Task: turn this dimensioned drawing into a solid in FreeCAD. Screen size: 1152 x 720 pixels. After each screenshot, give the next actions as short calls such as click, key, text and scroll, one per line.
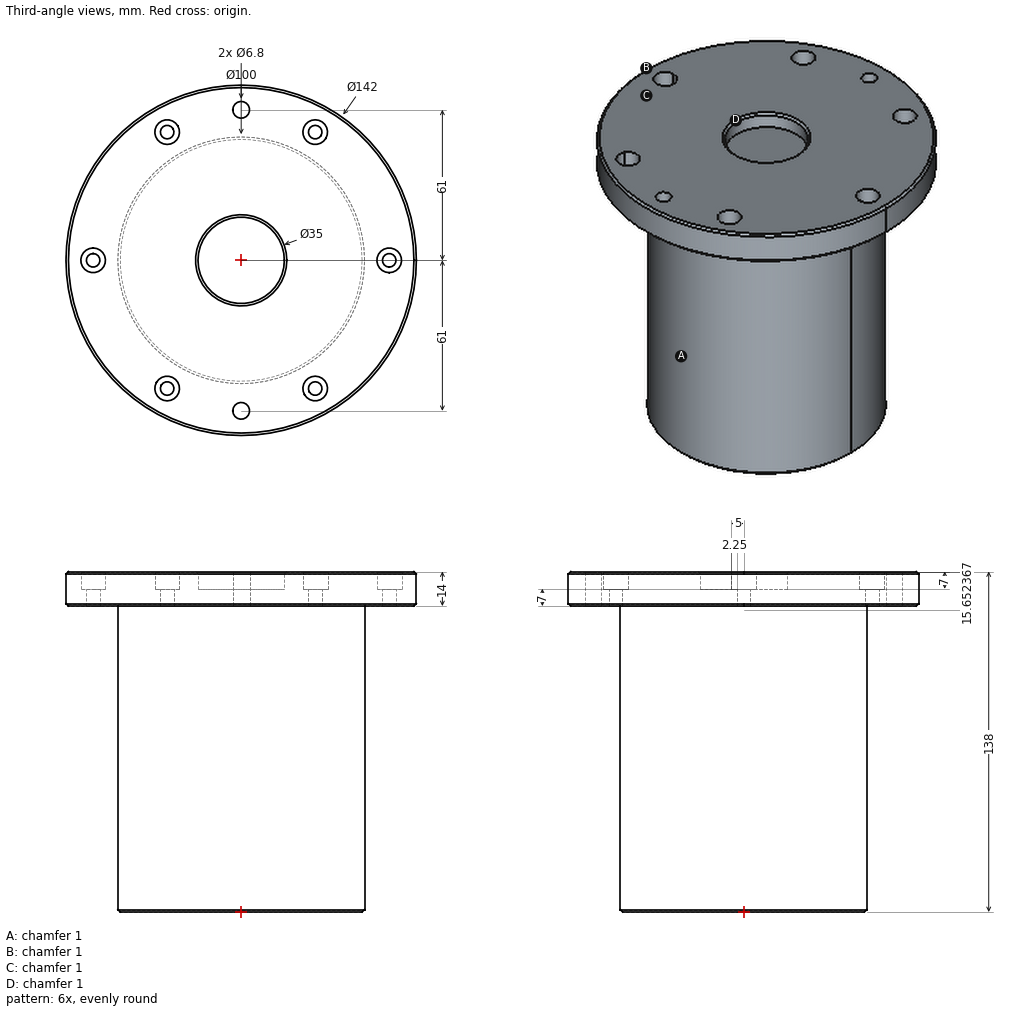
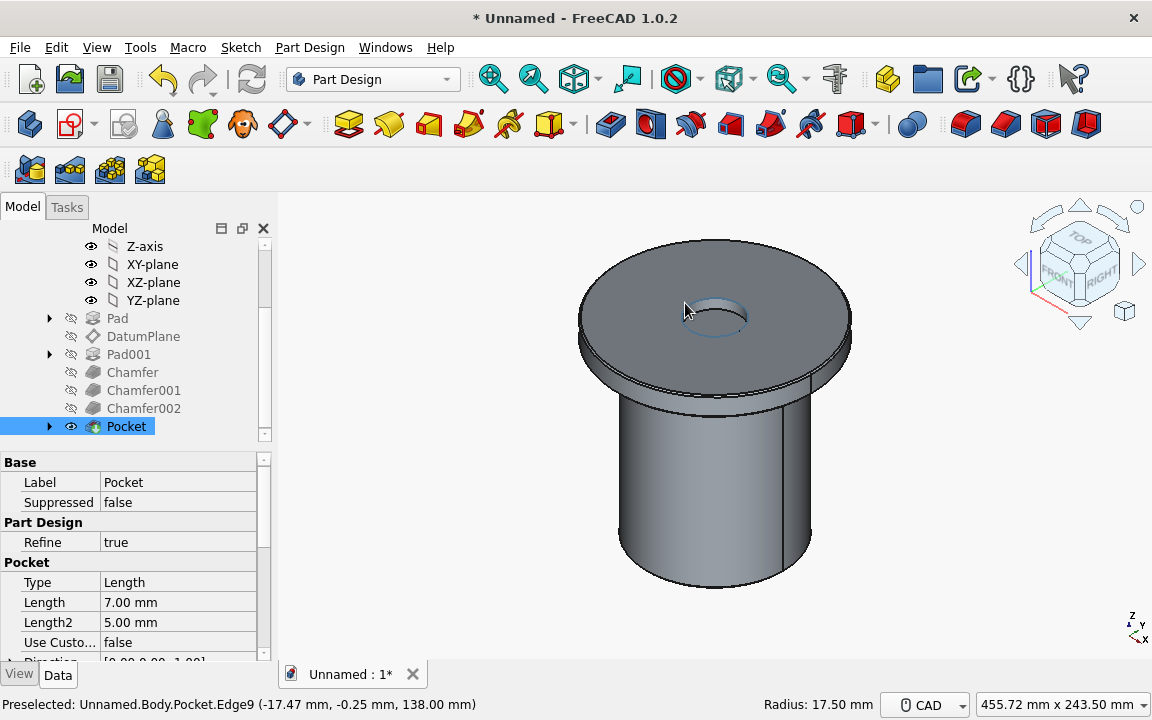
click(1006, 124)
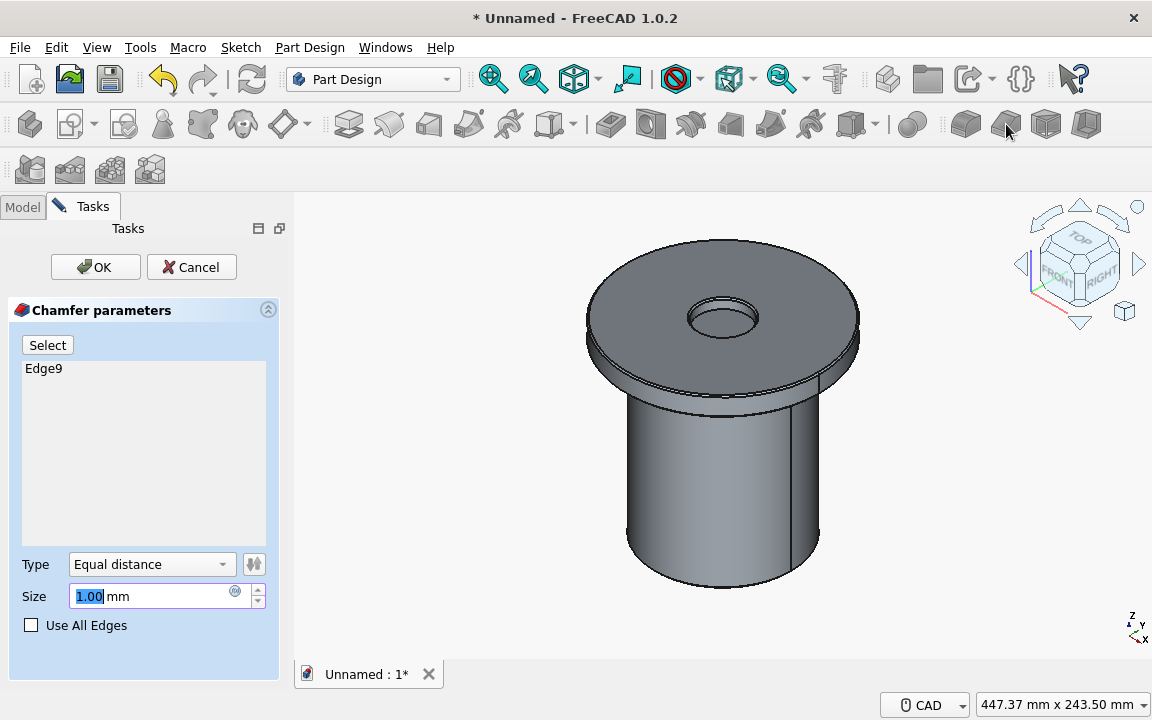
text(1)
key(Tab)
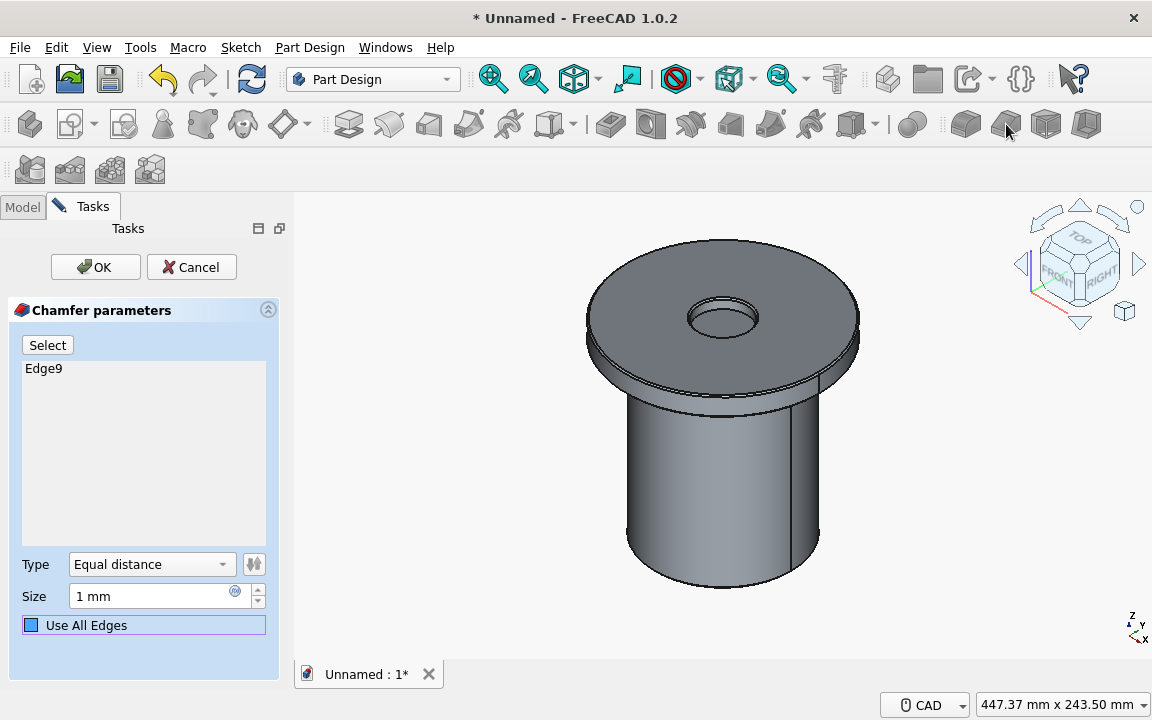
click(96, 267)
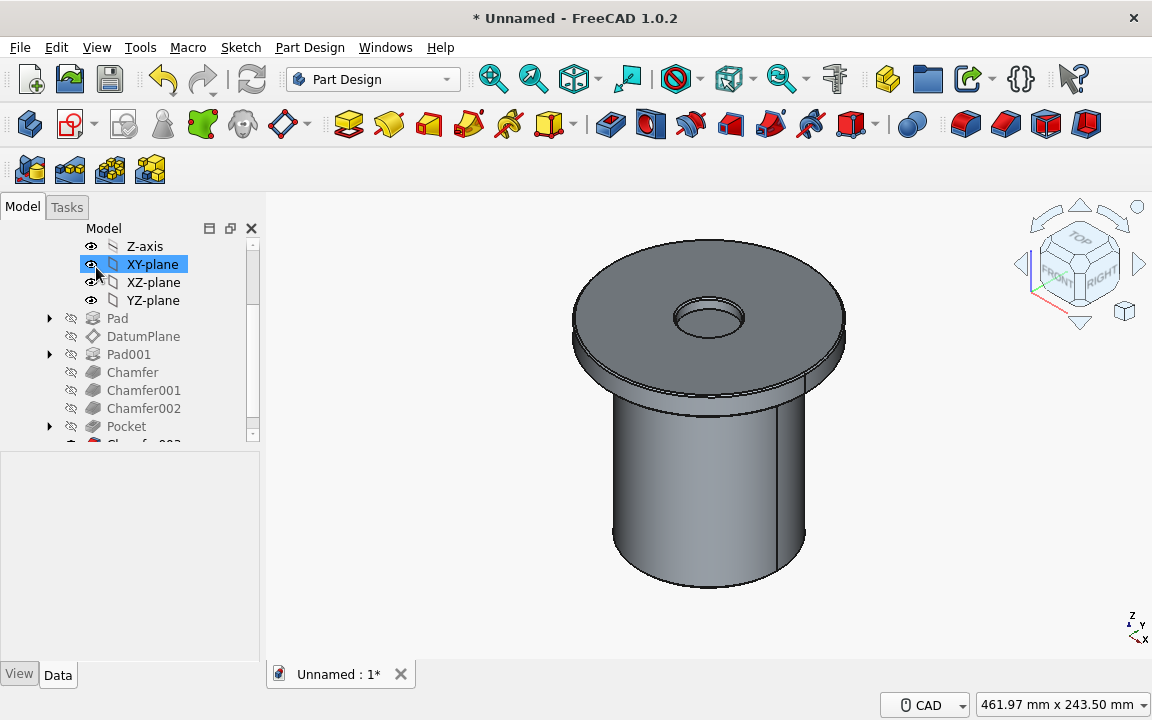
scroll(160, 332, down, 3)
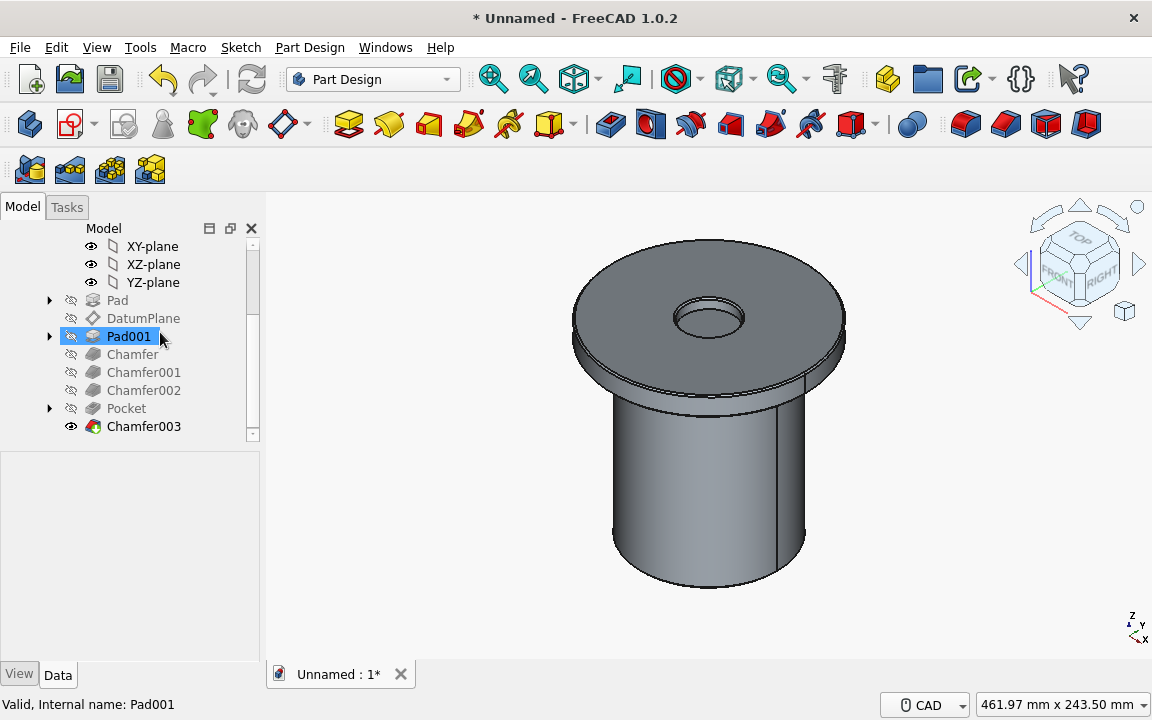
scroll(160, 332, up, 15)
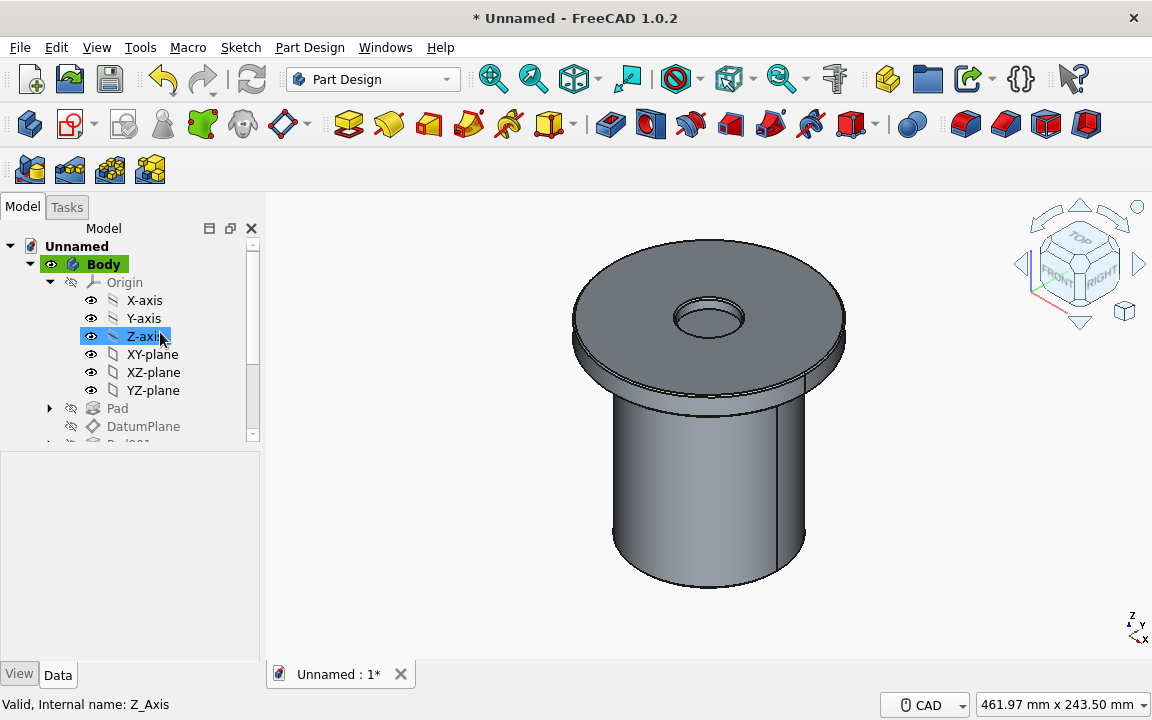
click(136, 390)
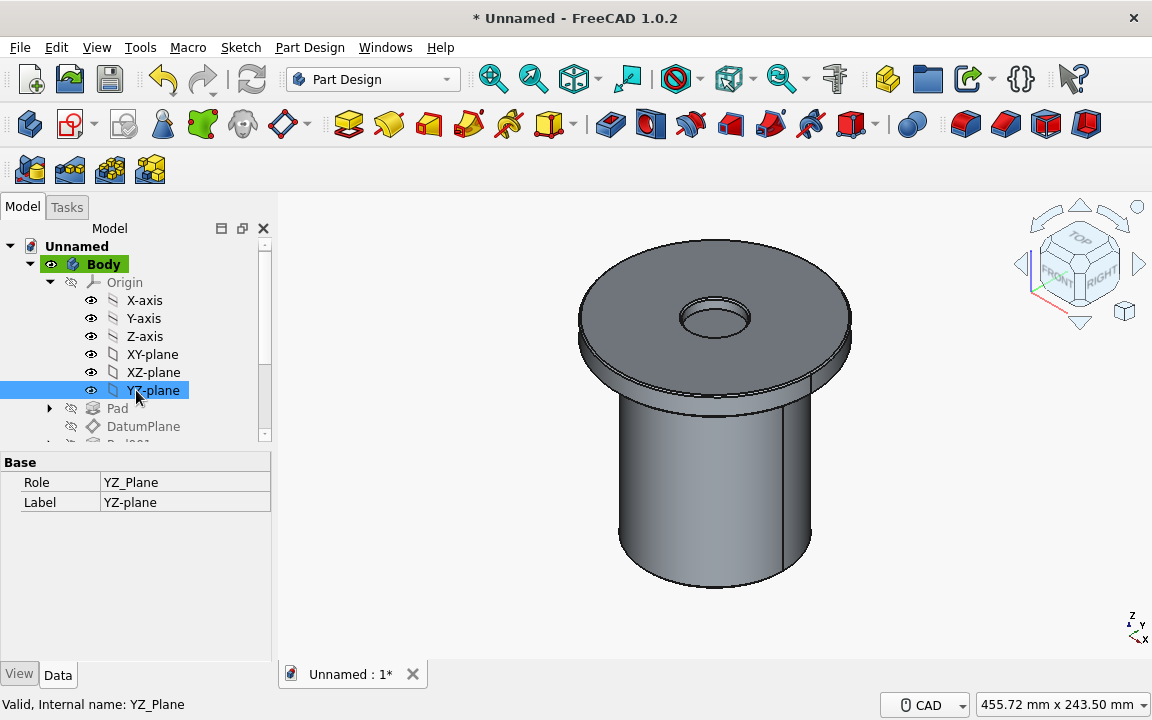
click(284, 124)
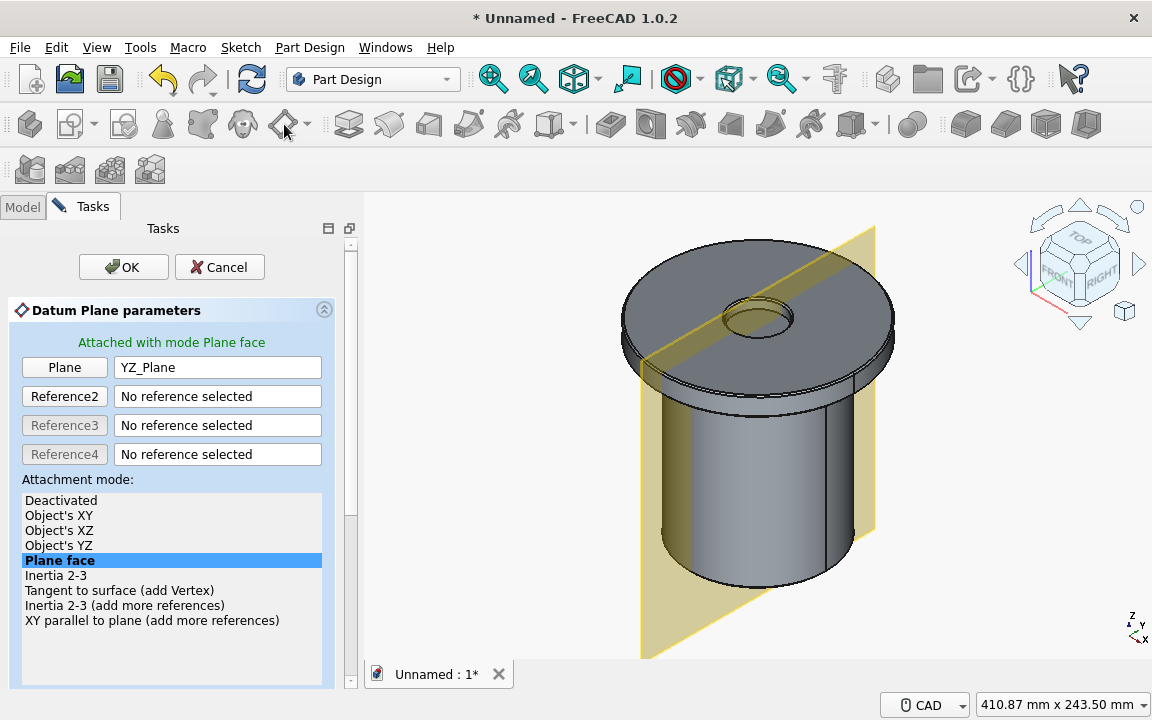
scroll(351, 463, down, 3)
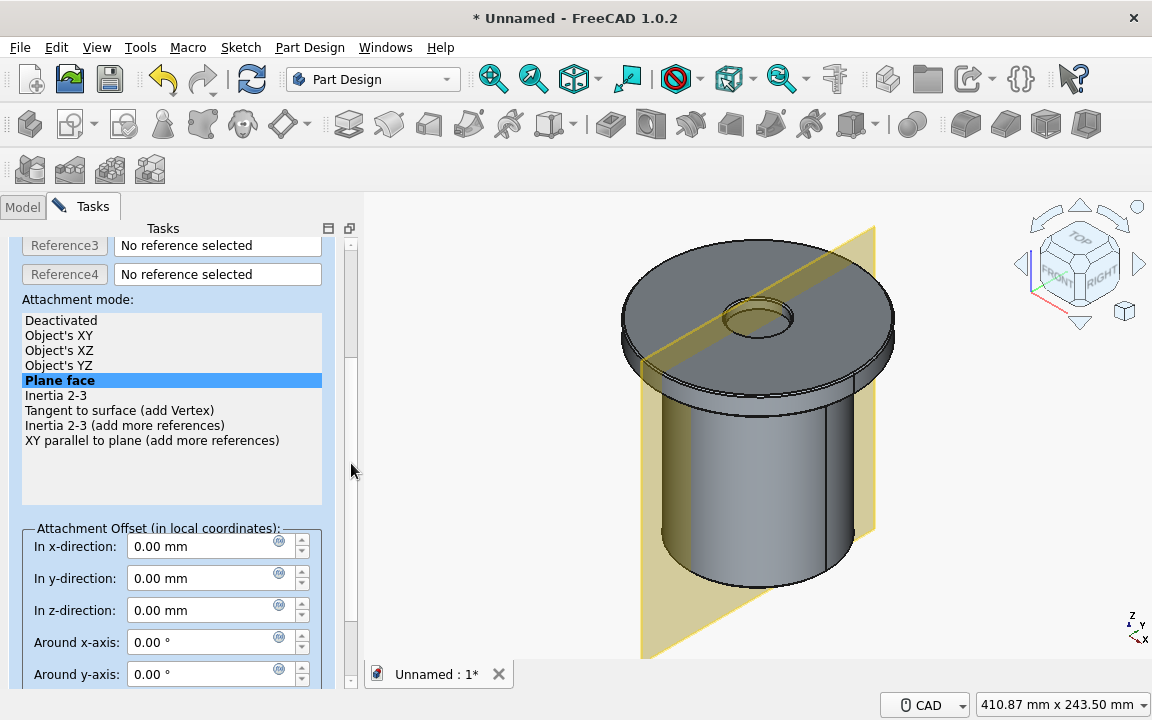
triple_click(210, 610)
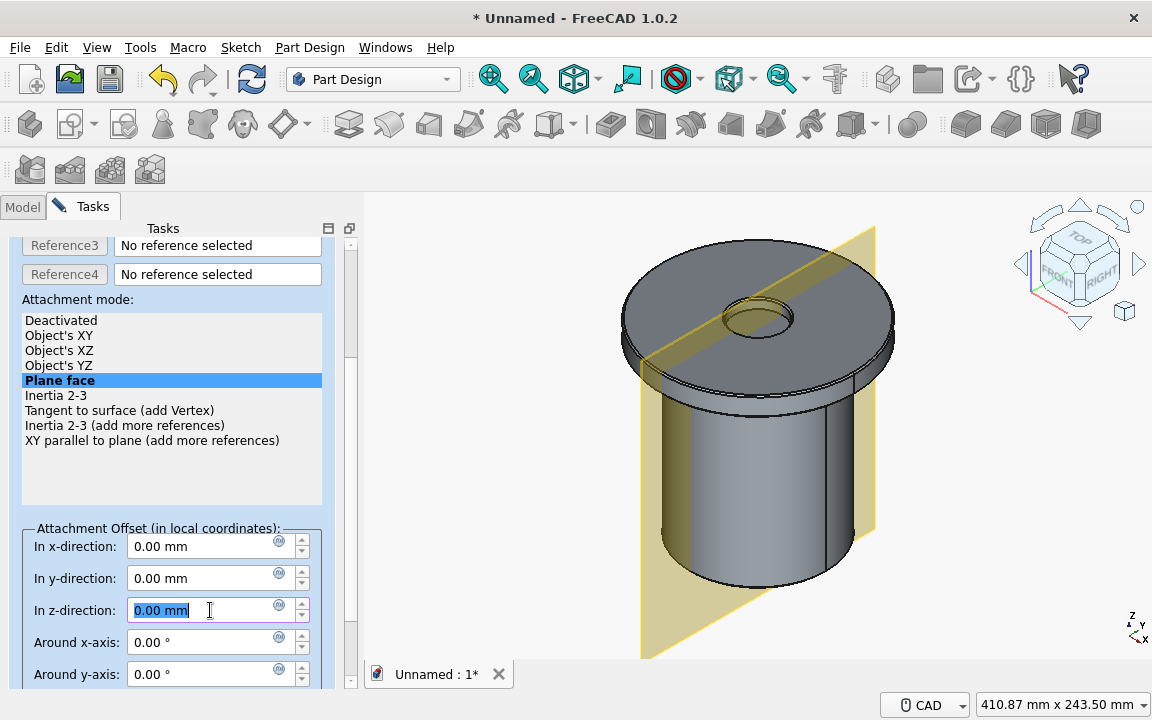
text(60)
key(Tab)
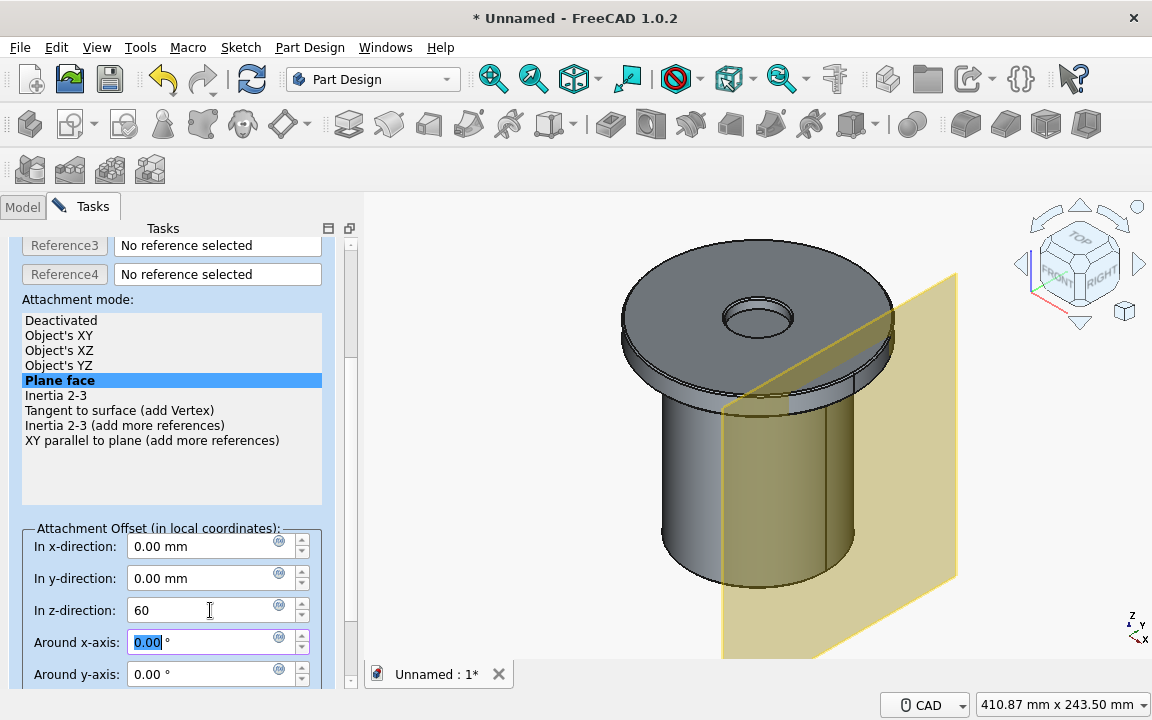
scroll(351, 463, up, 4)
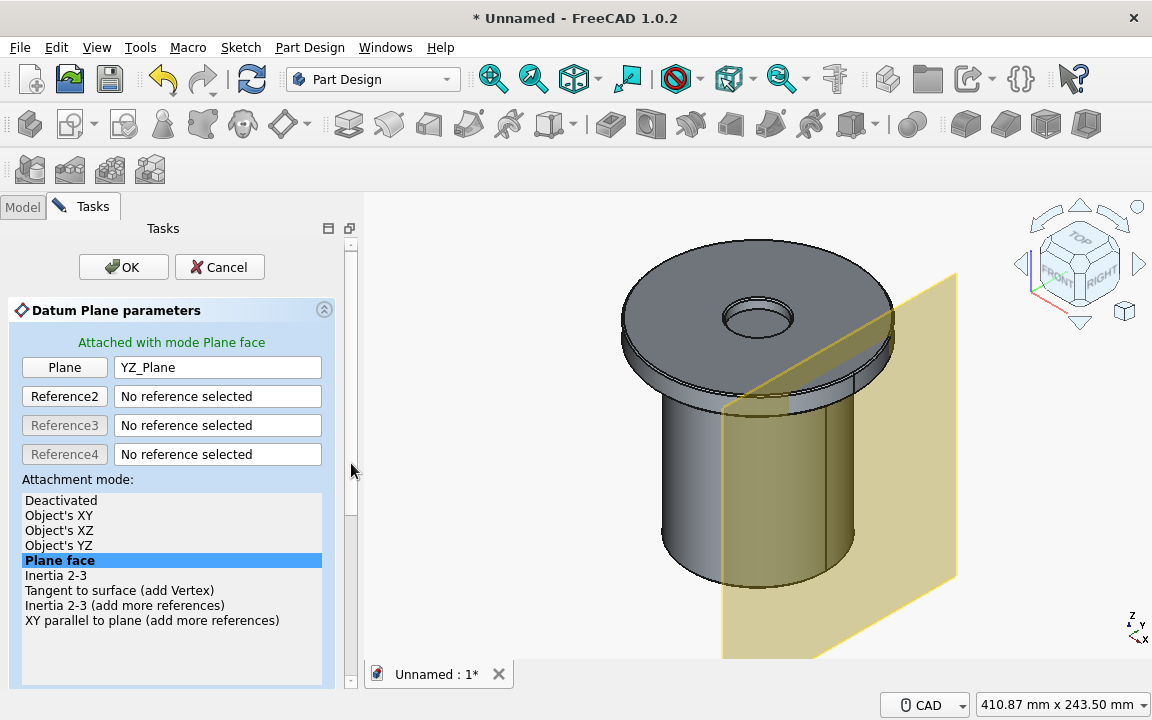
click(124, 267)